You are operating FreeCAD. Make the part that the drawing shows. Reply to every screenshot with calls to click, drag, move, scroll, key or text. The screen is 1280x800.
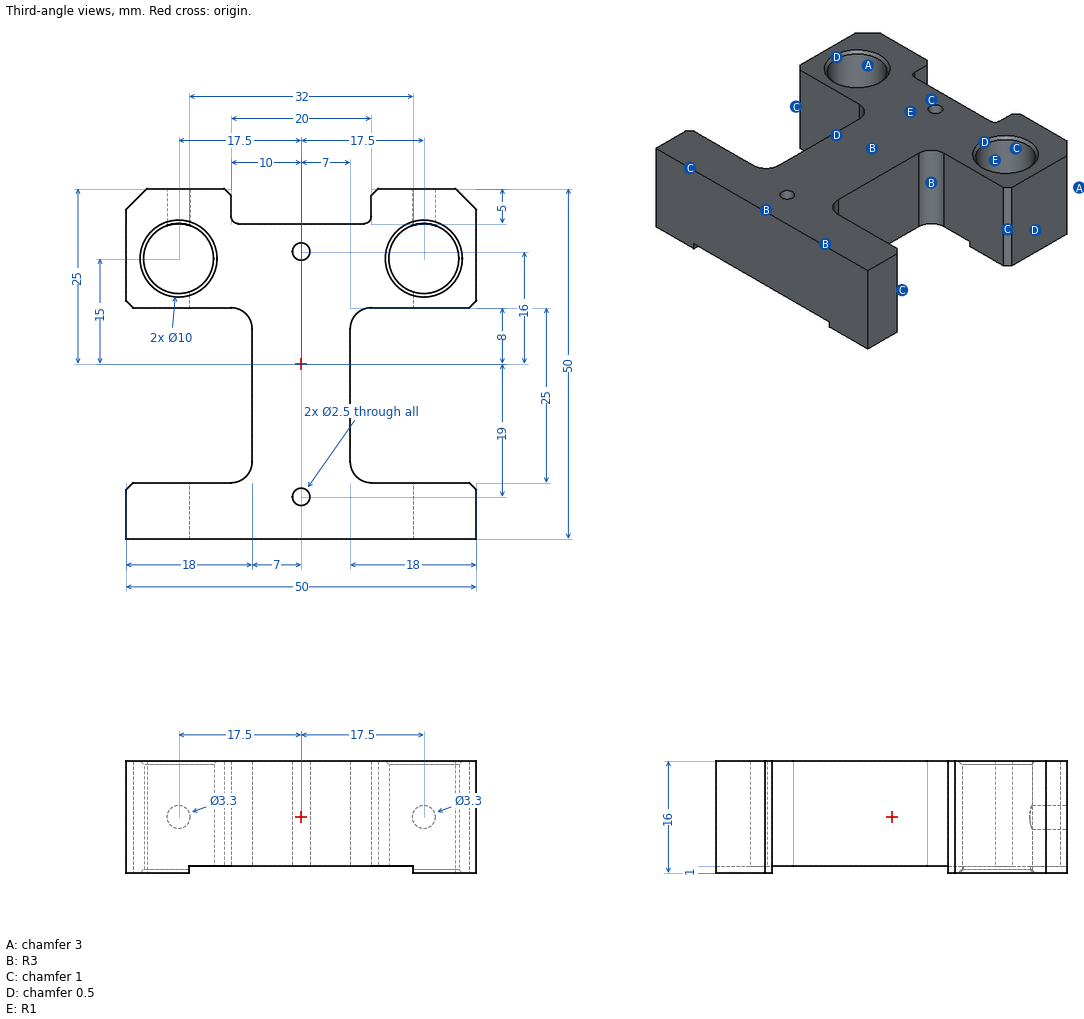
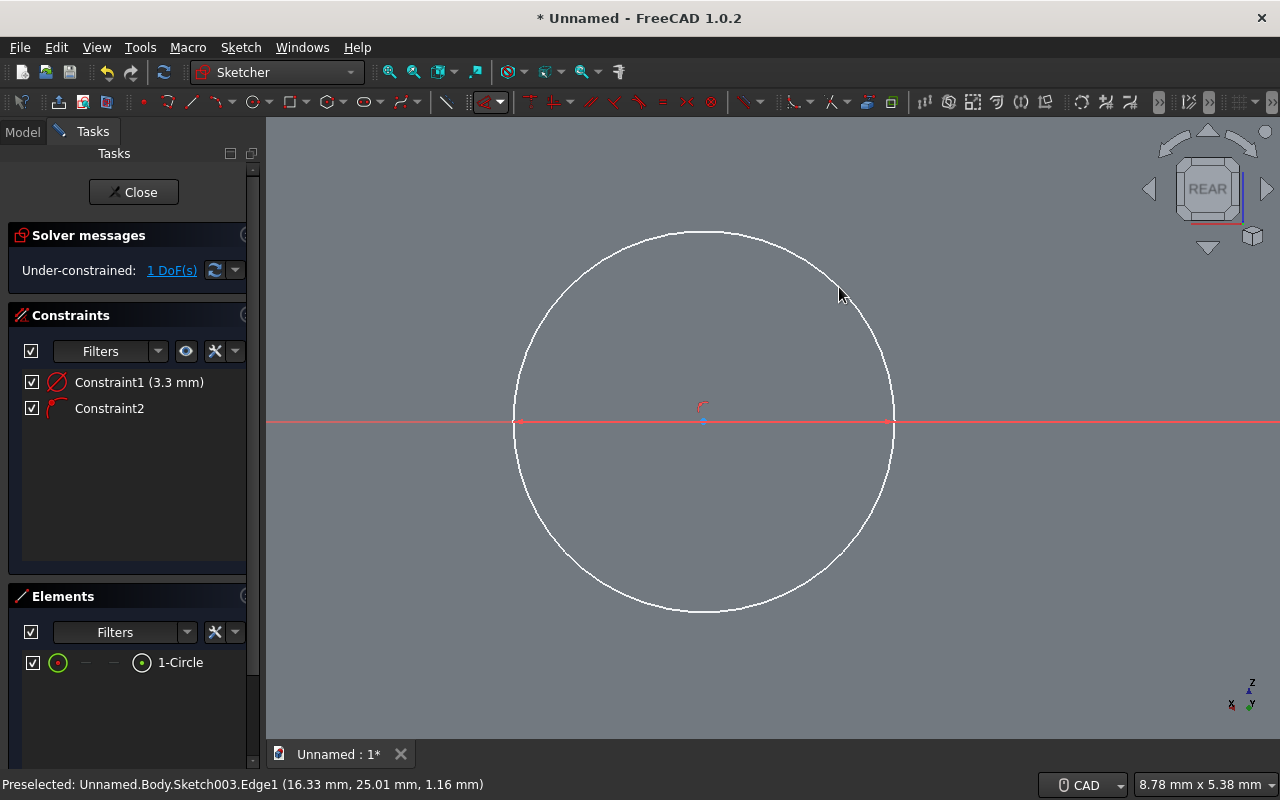
click(484, 102)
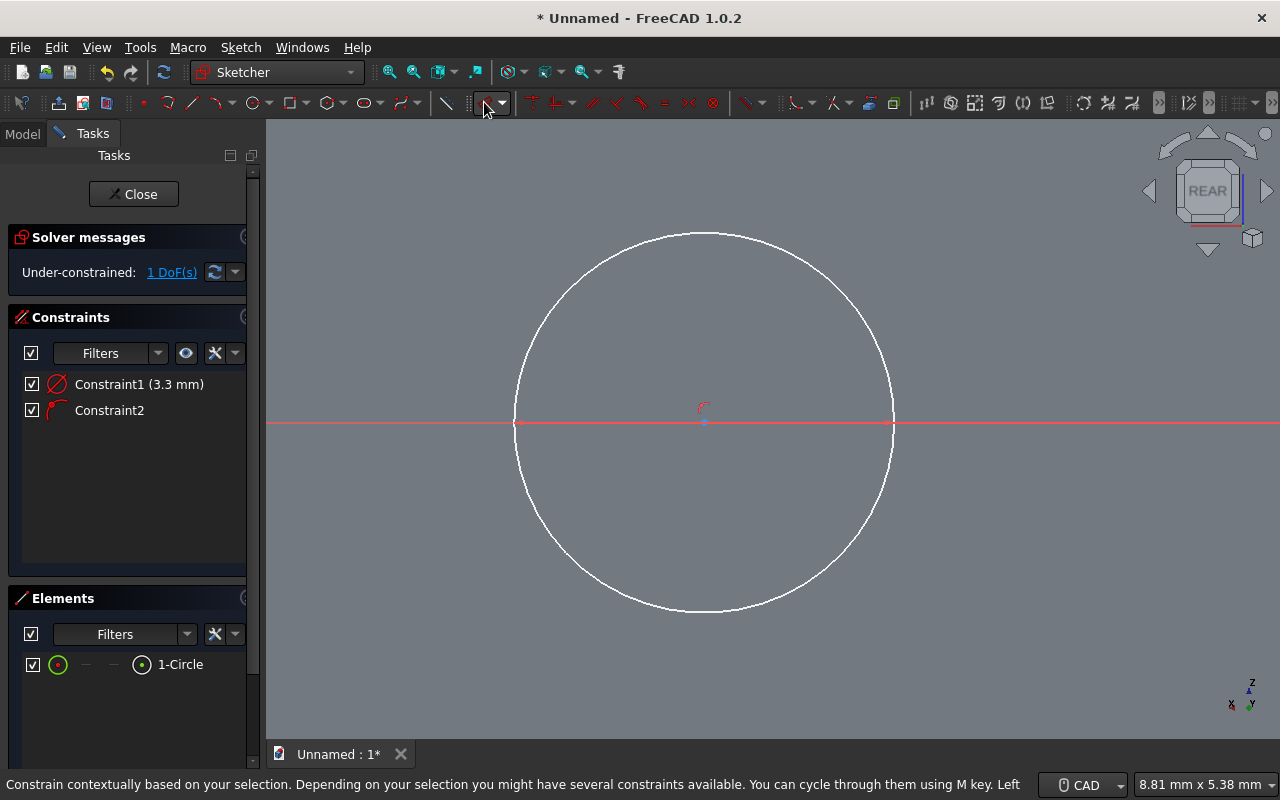
click(704, 423)
click(910, 457)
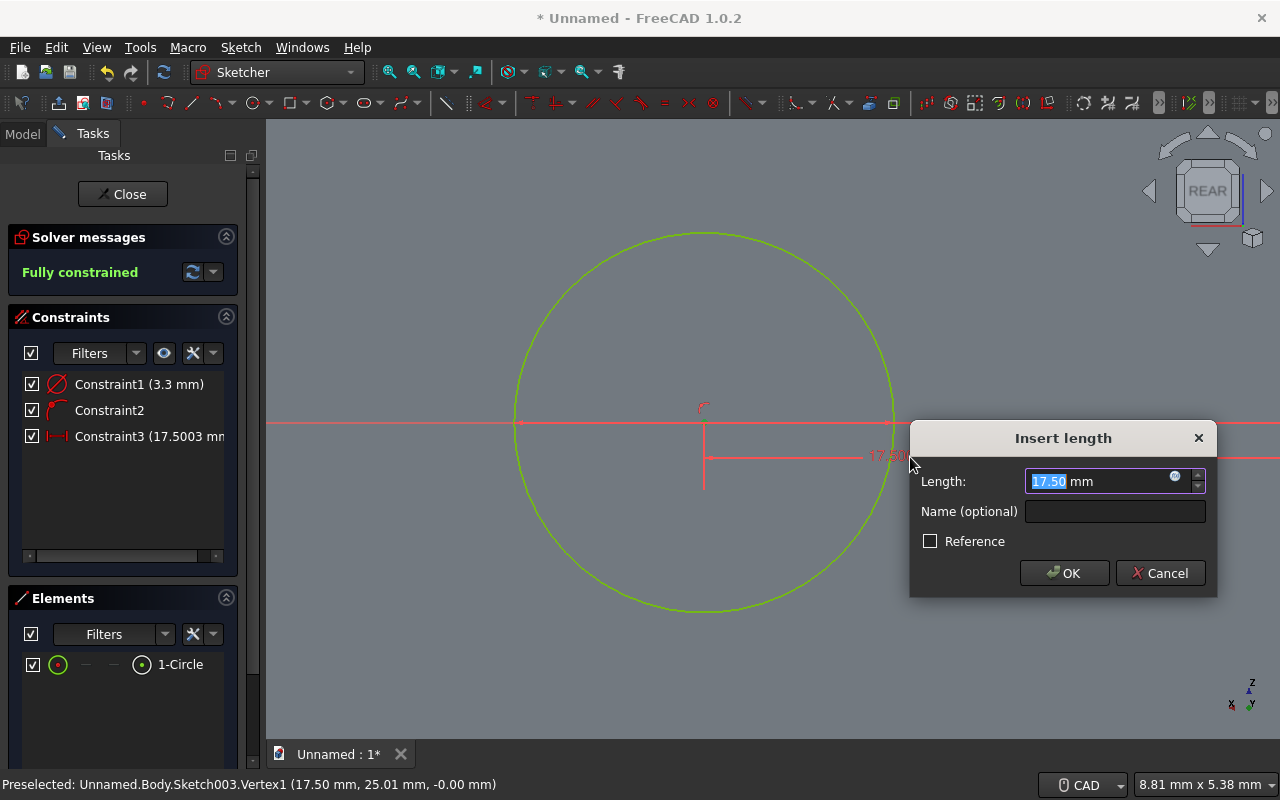
text(17.5)
key(Return)
key(Escape)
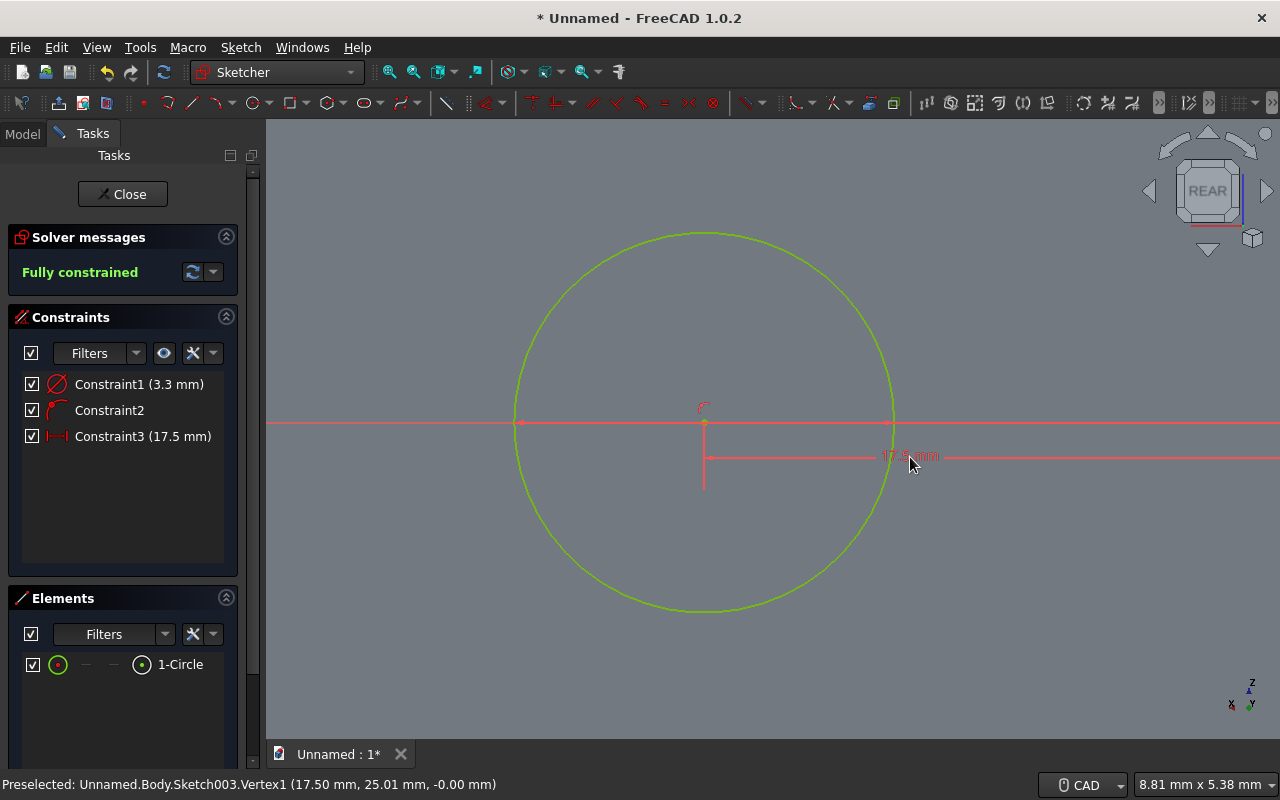
click(123, 194)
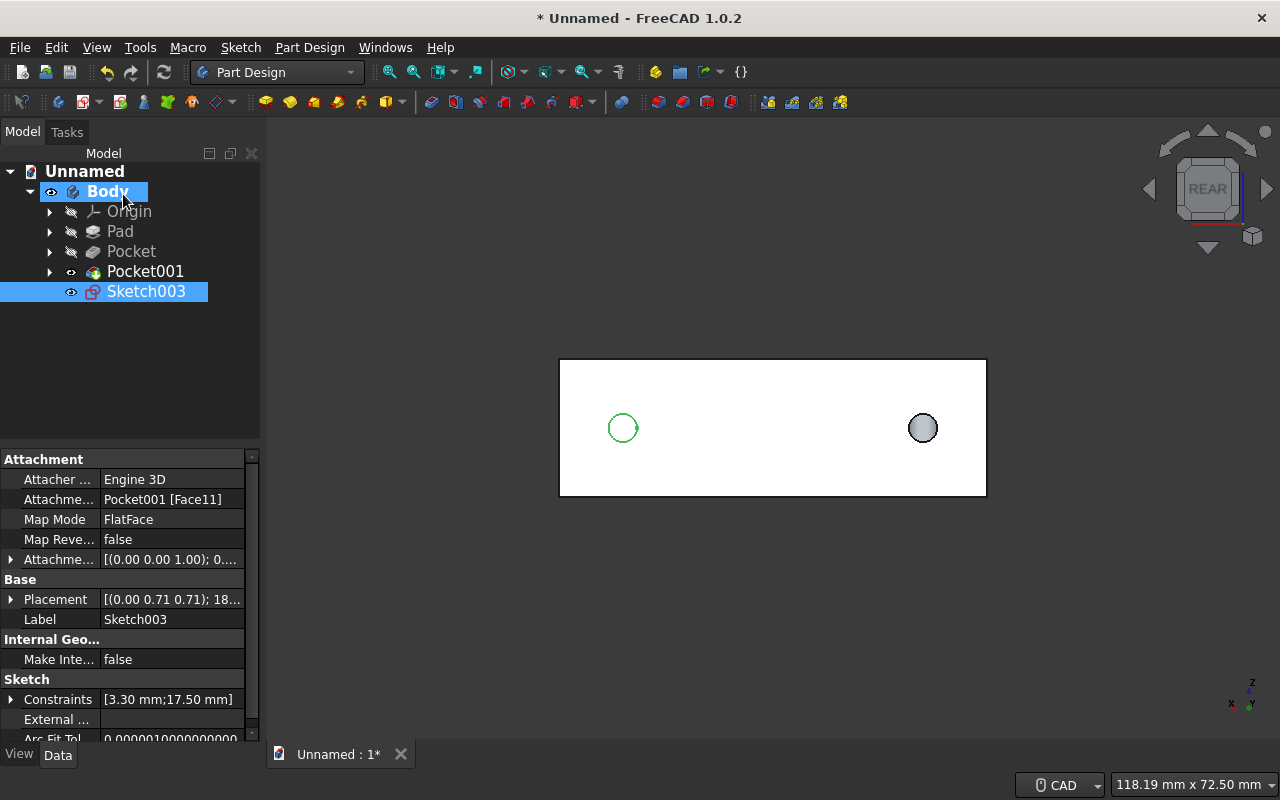
click(432, 102)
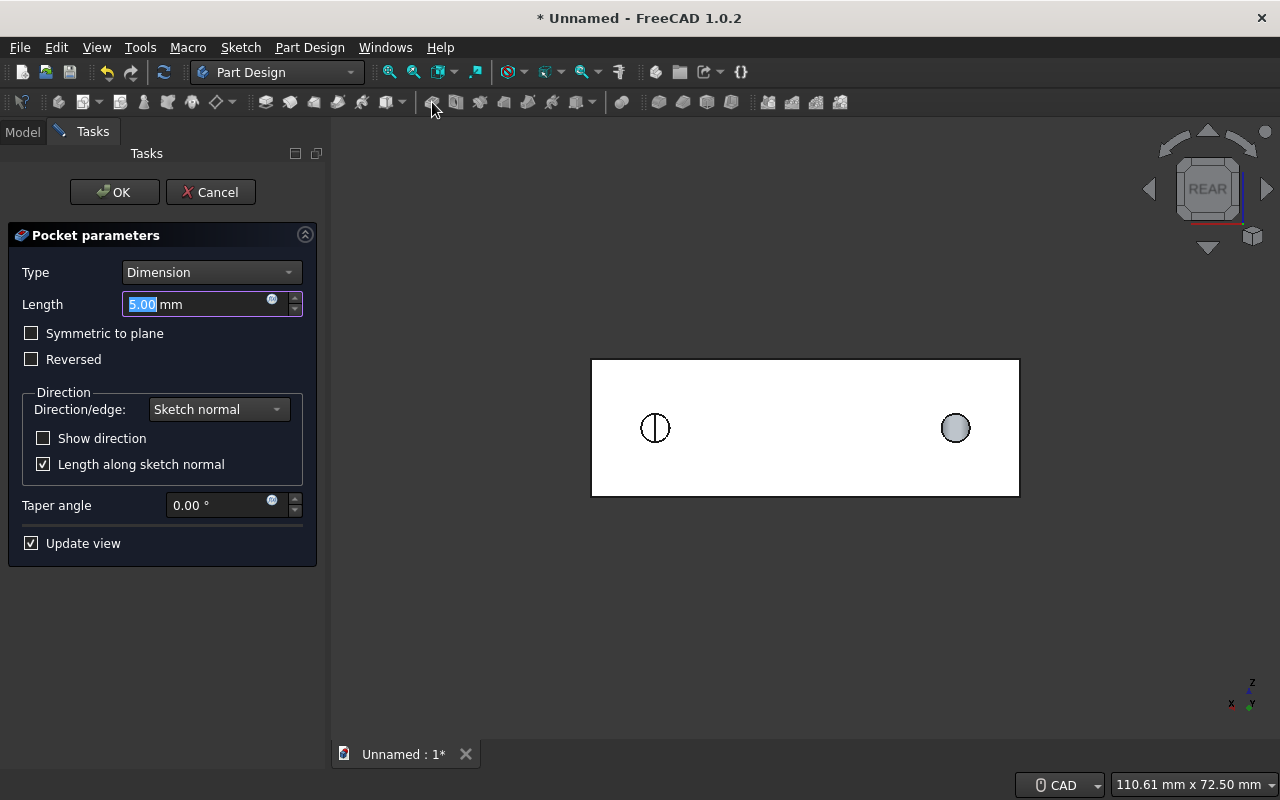
click(212, 272)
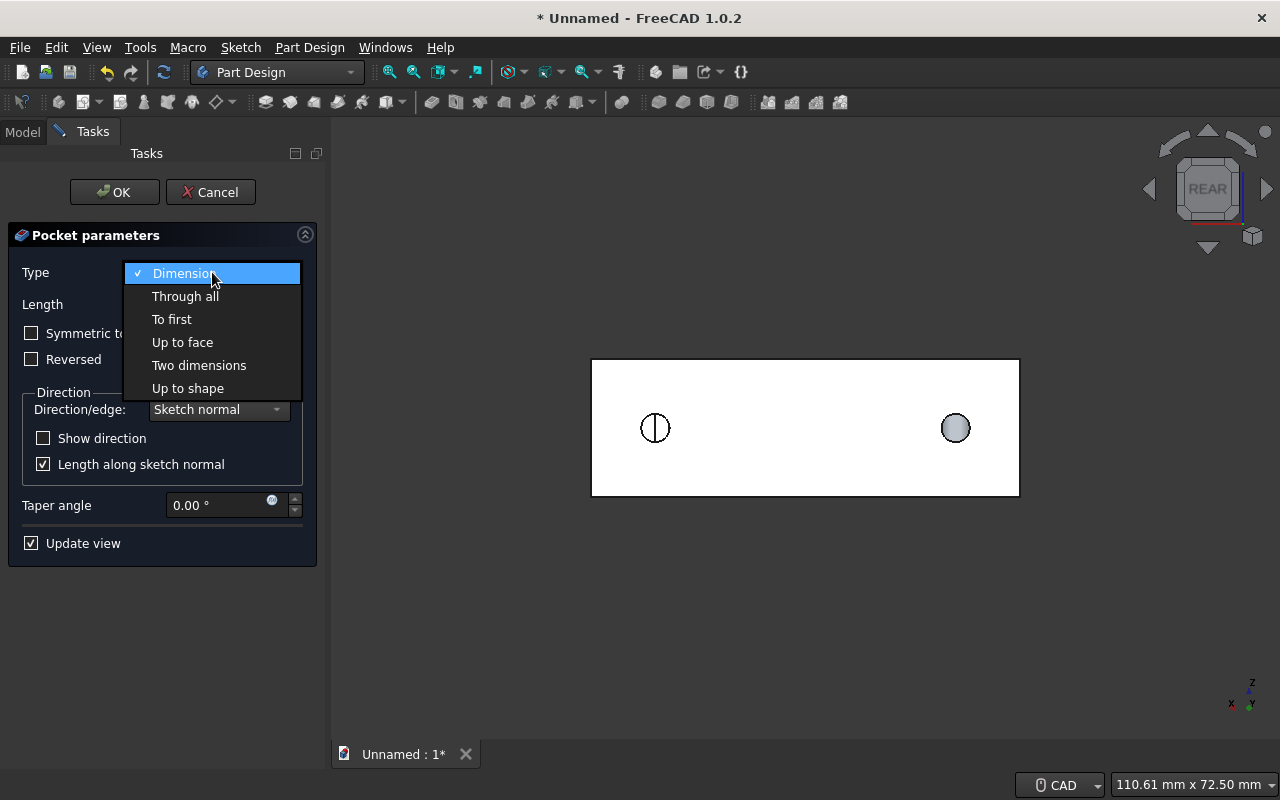
click(212, 320)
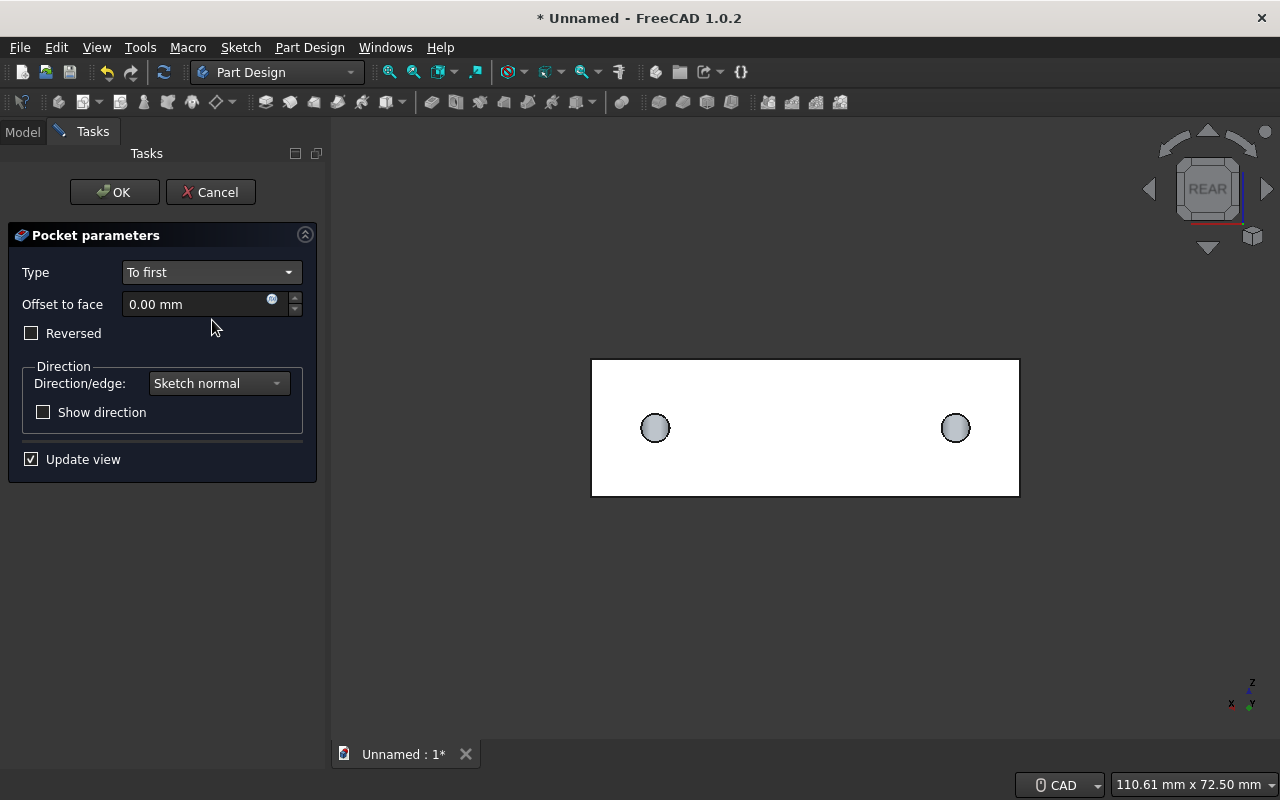
click(115, 192)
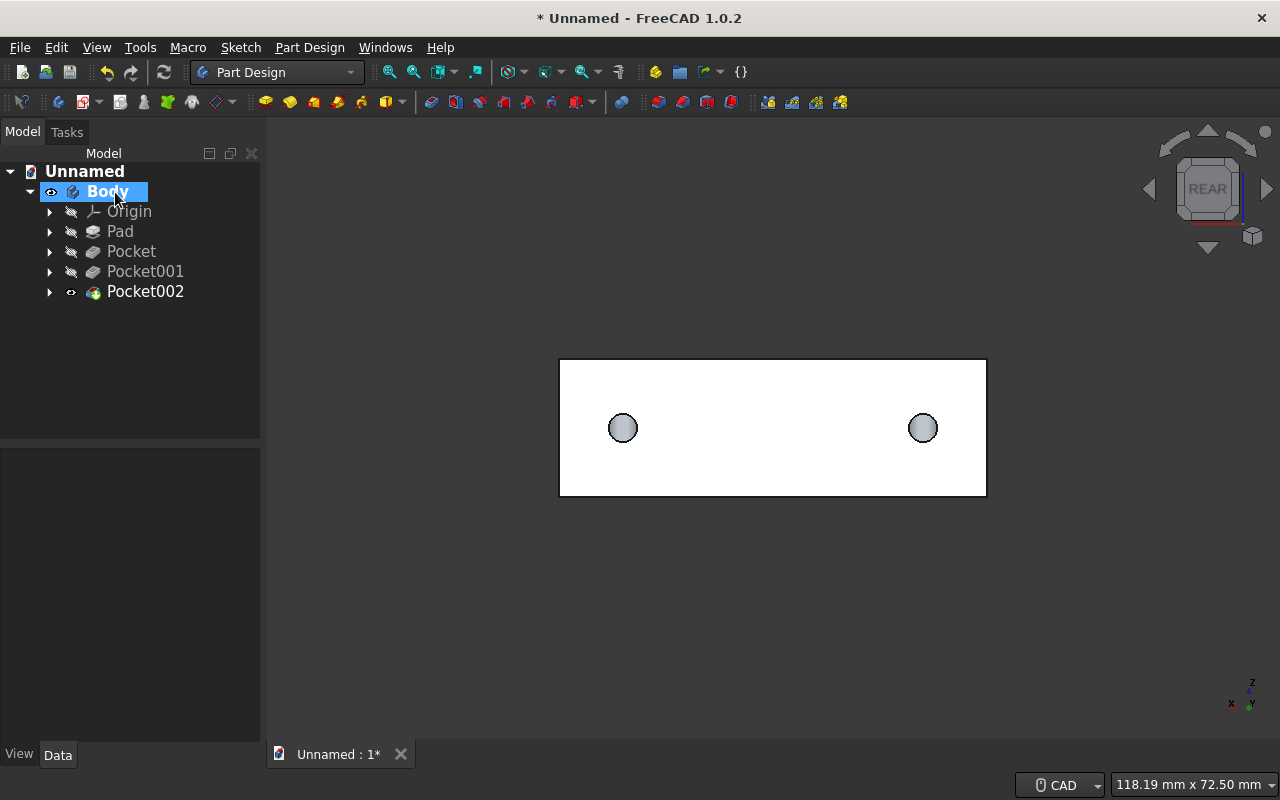
key(v)
key(f)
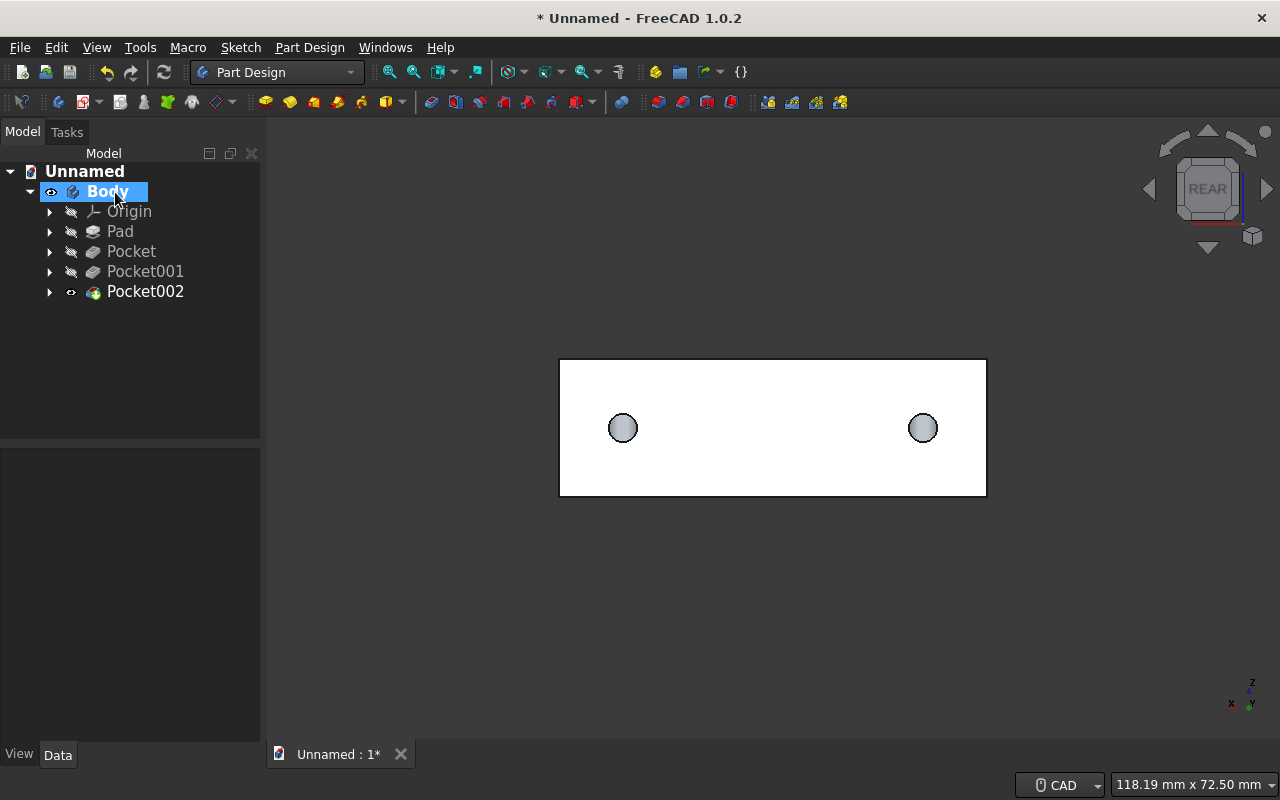
key(0)